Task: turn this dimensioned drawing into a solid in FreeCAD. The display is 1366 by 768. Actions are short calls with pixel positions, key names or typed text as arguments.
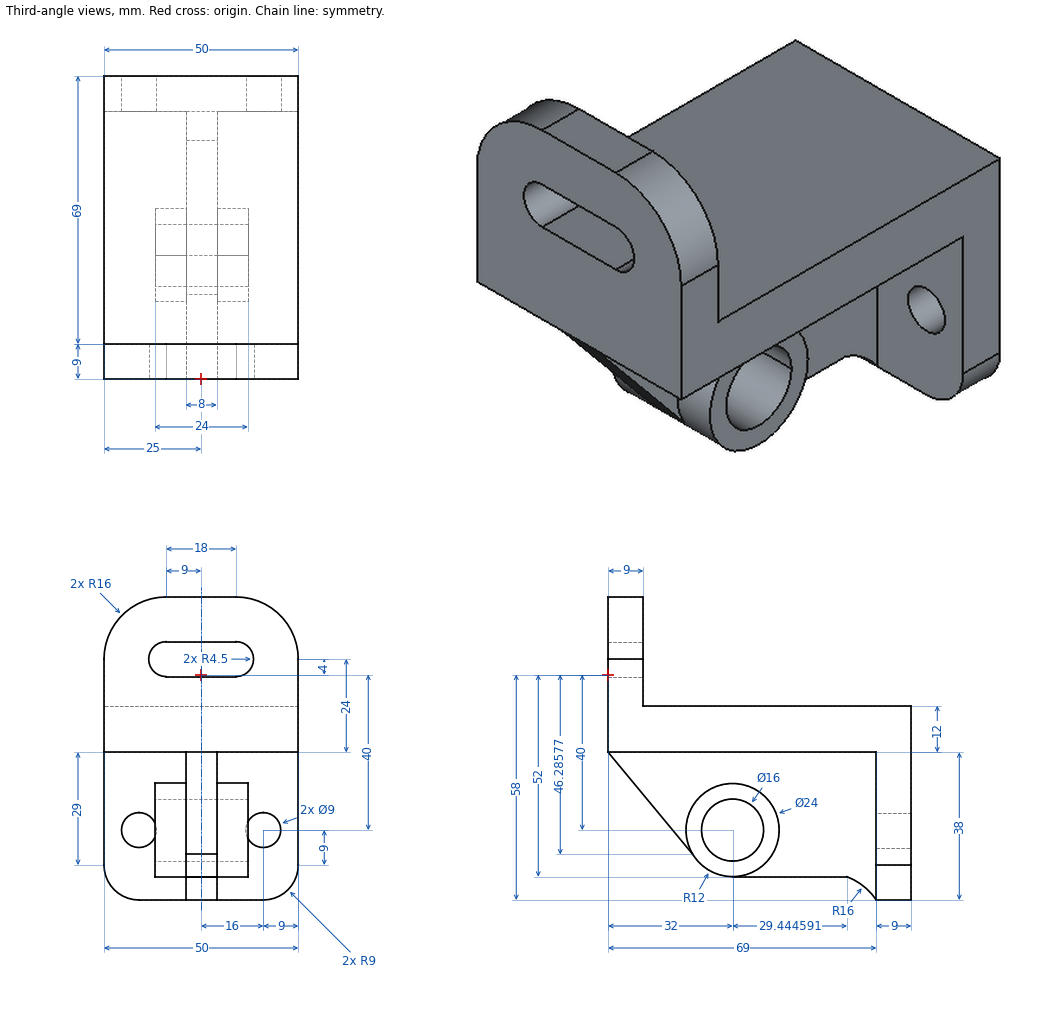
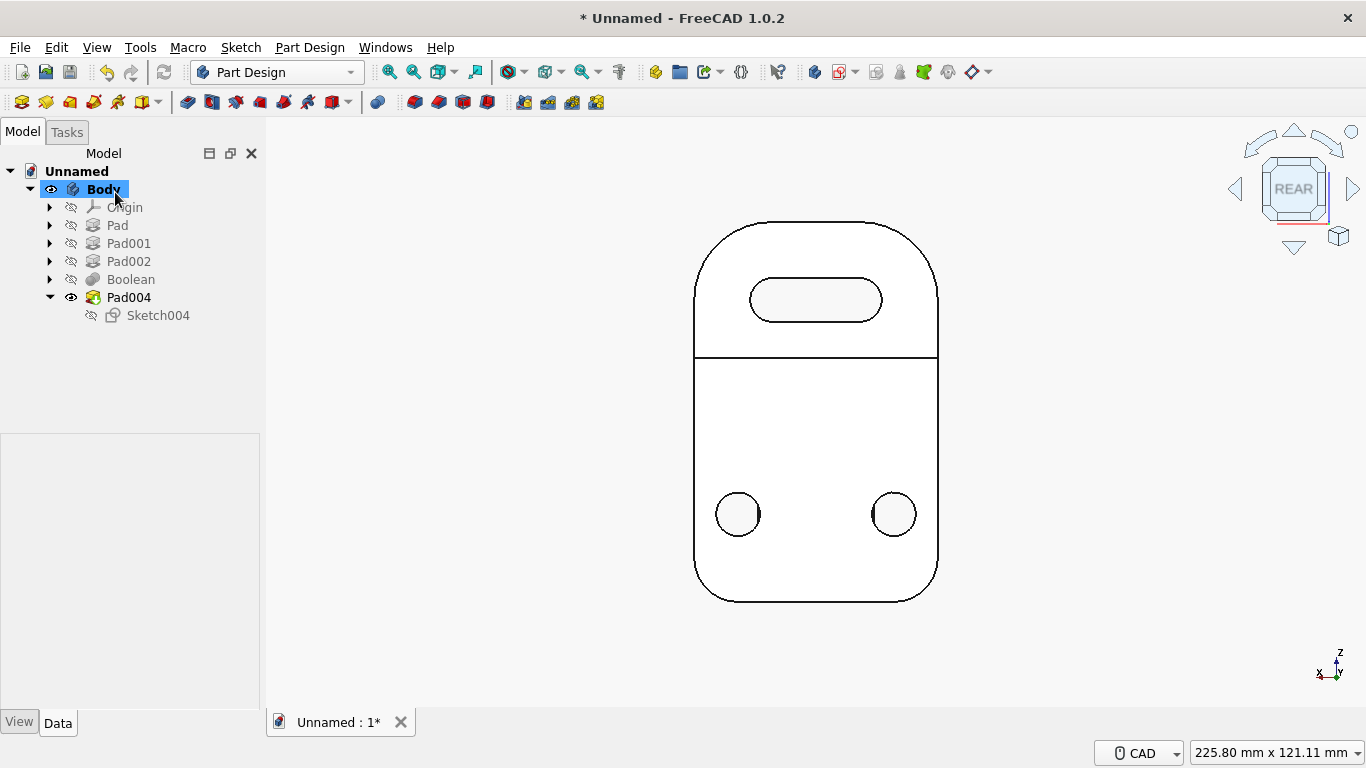
key(6)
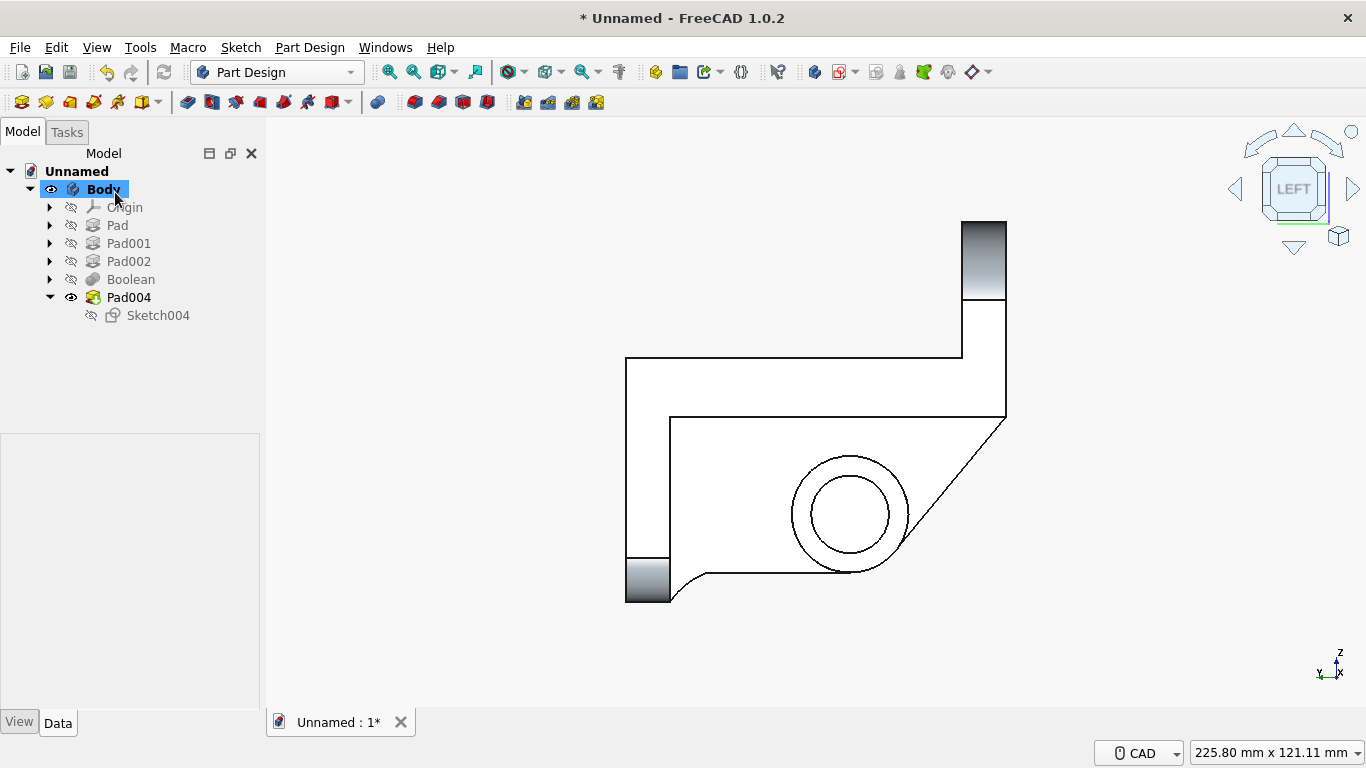
click(742, 482)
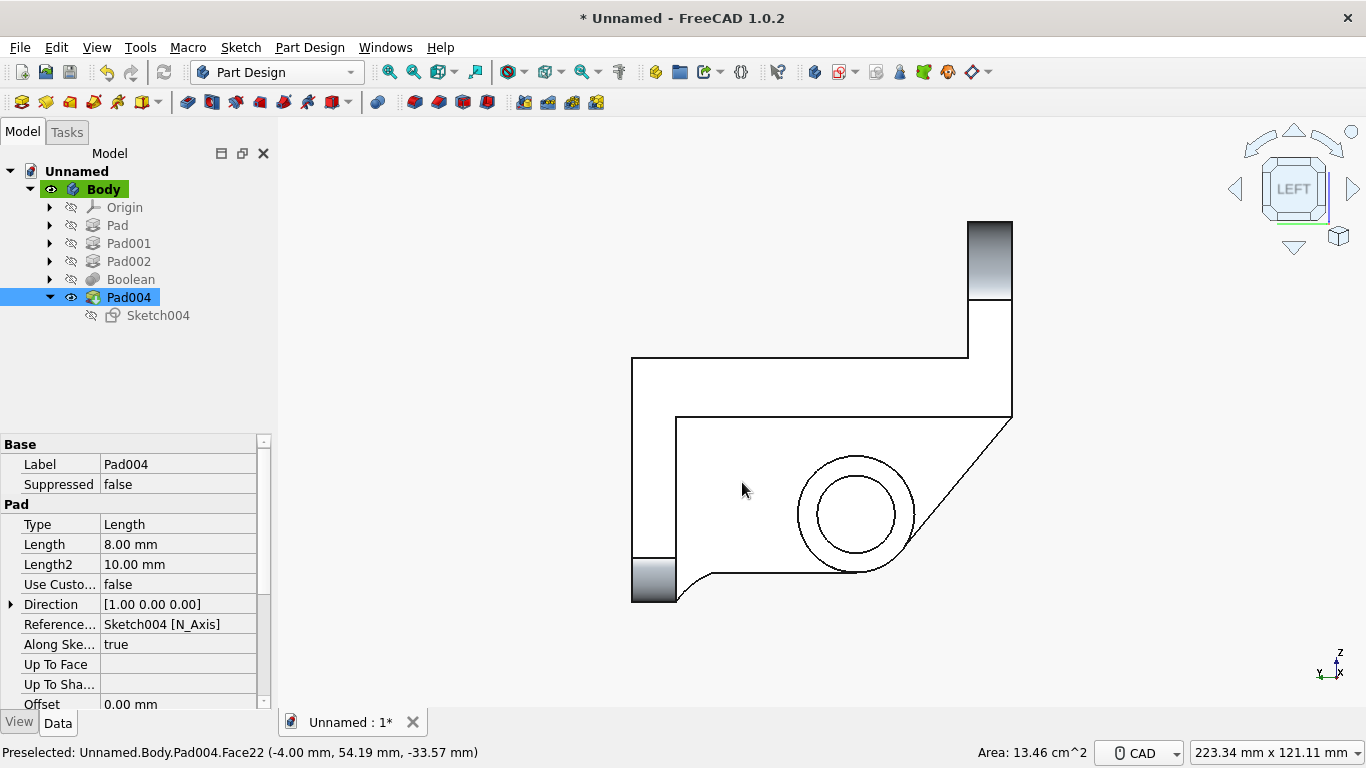
click(840, 72)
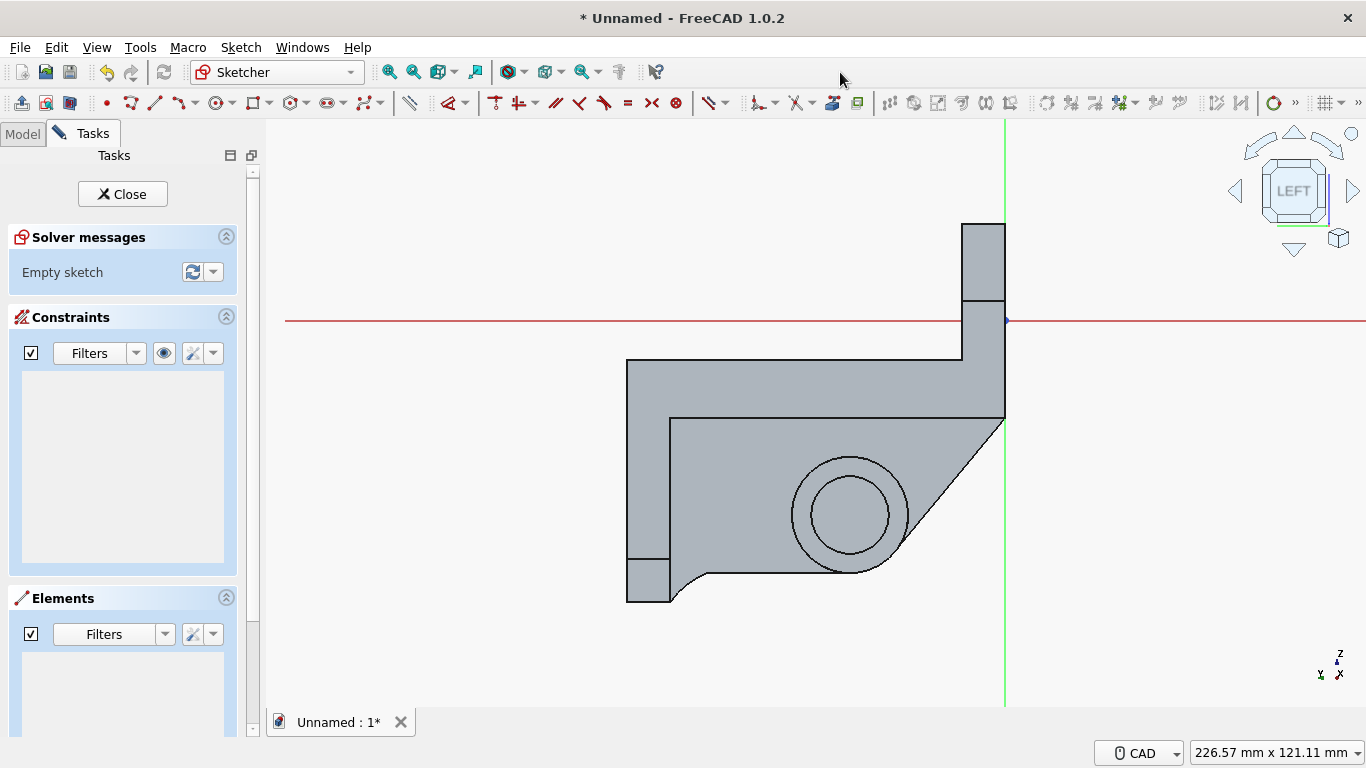
click(70, 104)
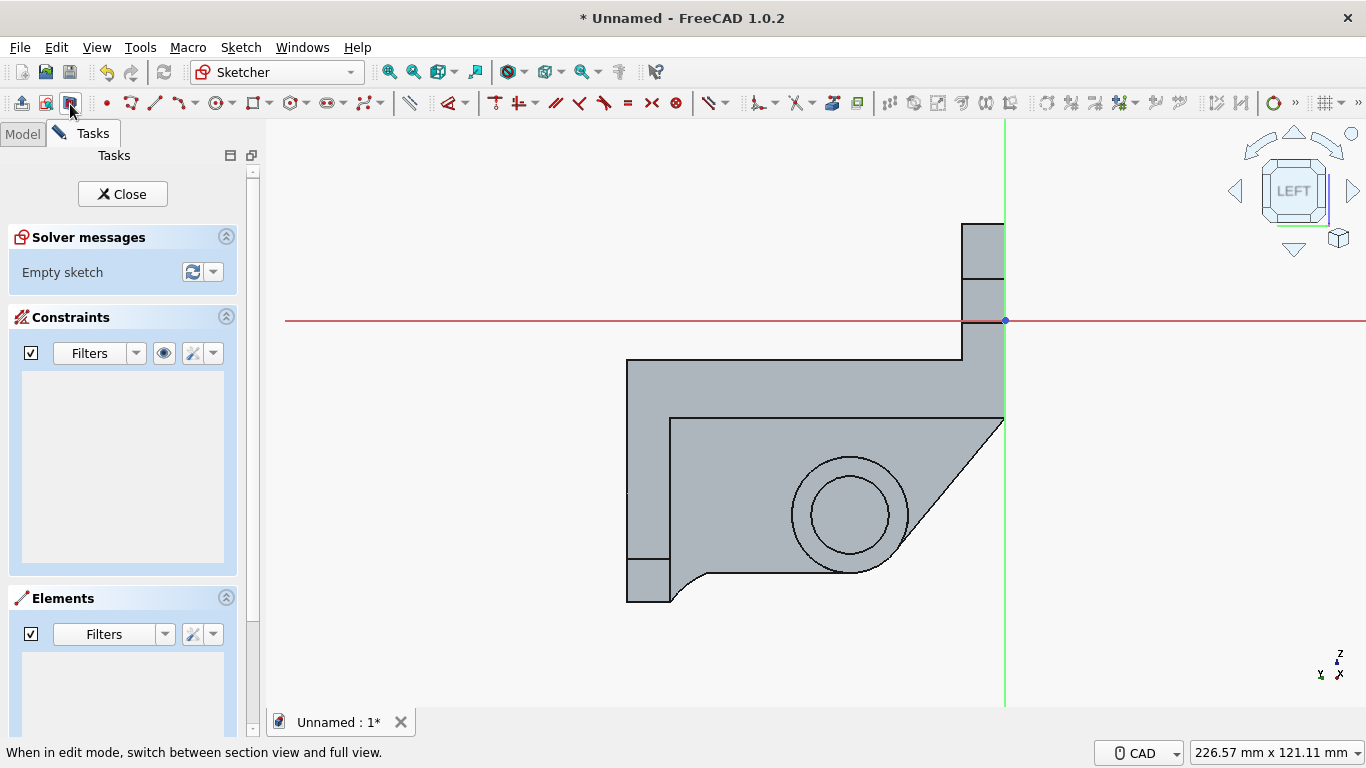
scroll(876, 541, up, 8)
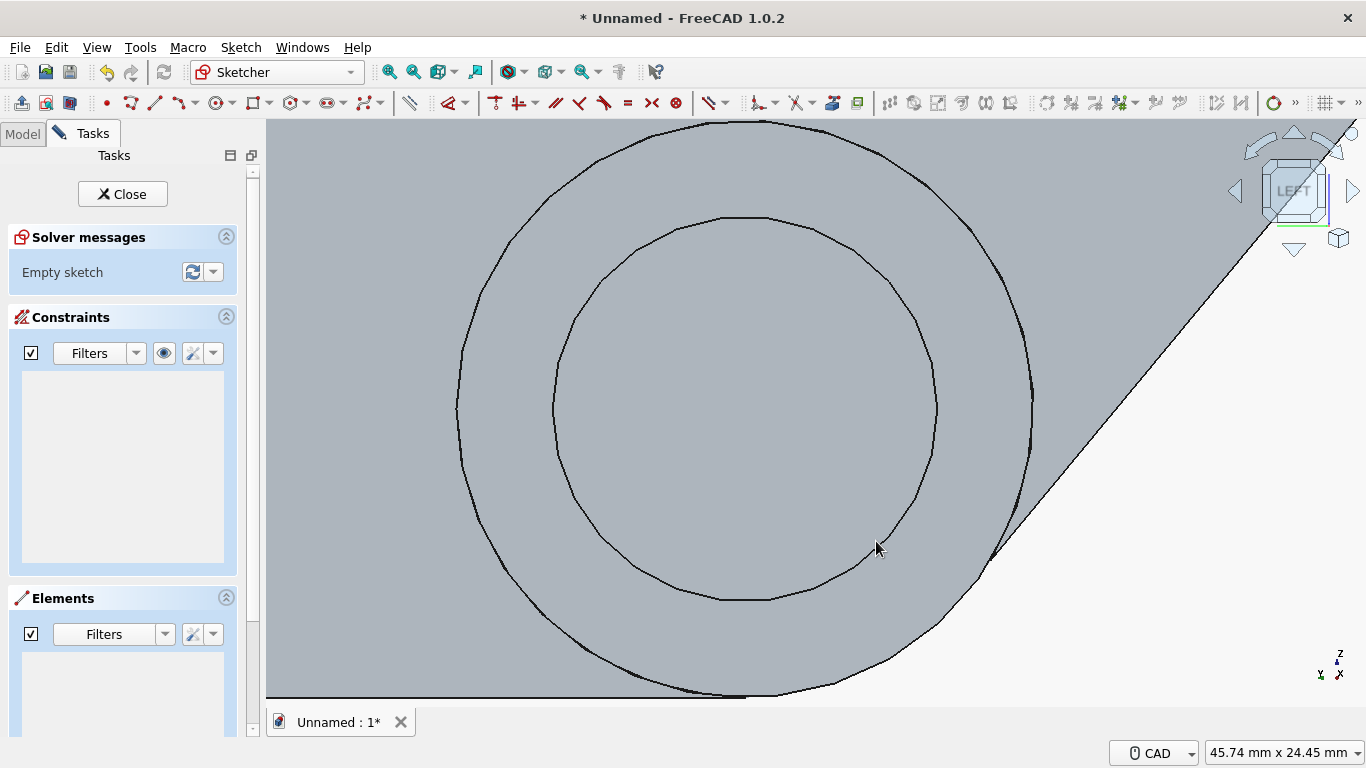
click(216, 104)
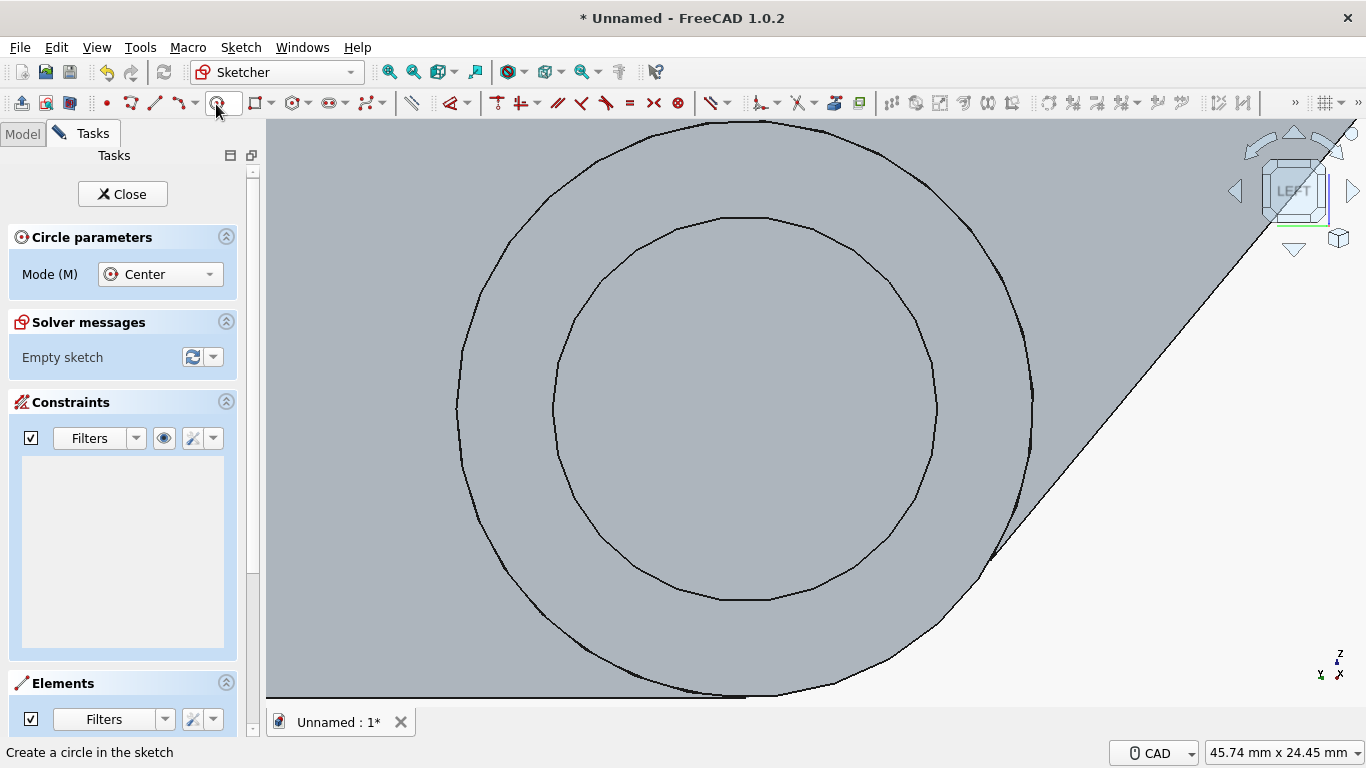
click(745, 409)
click(881, 273)
key(Escape)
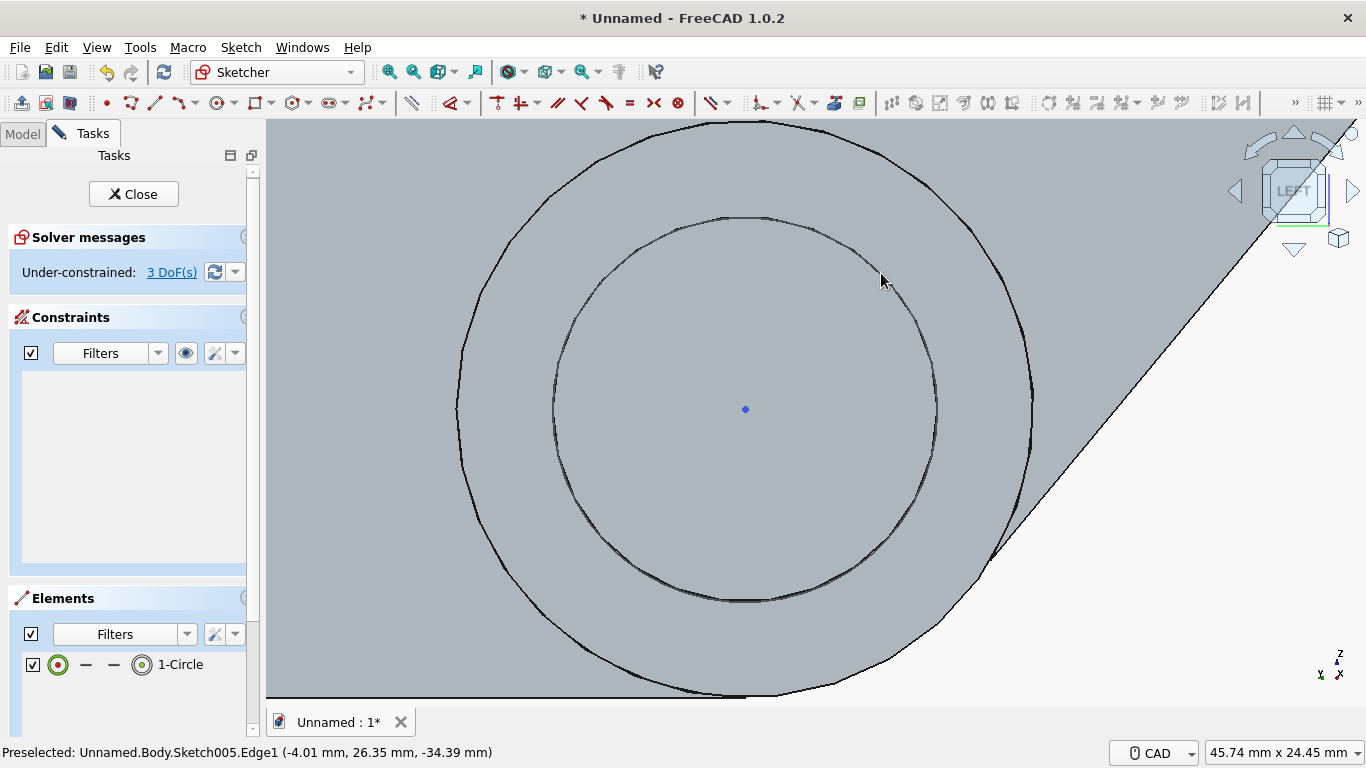
click(450, 104)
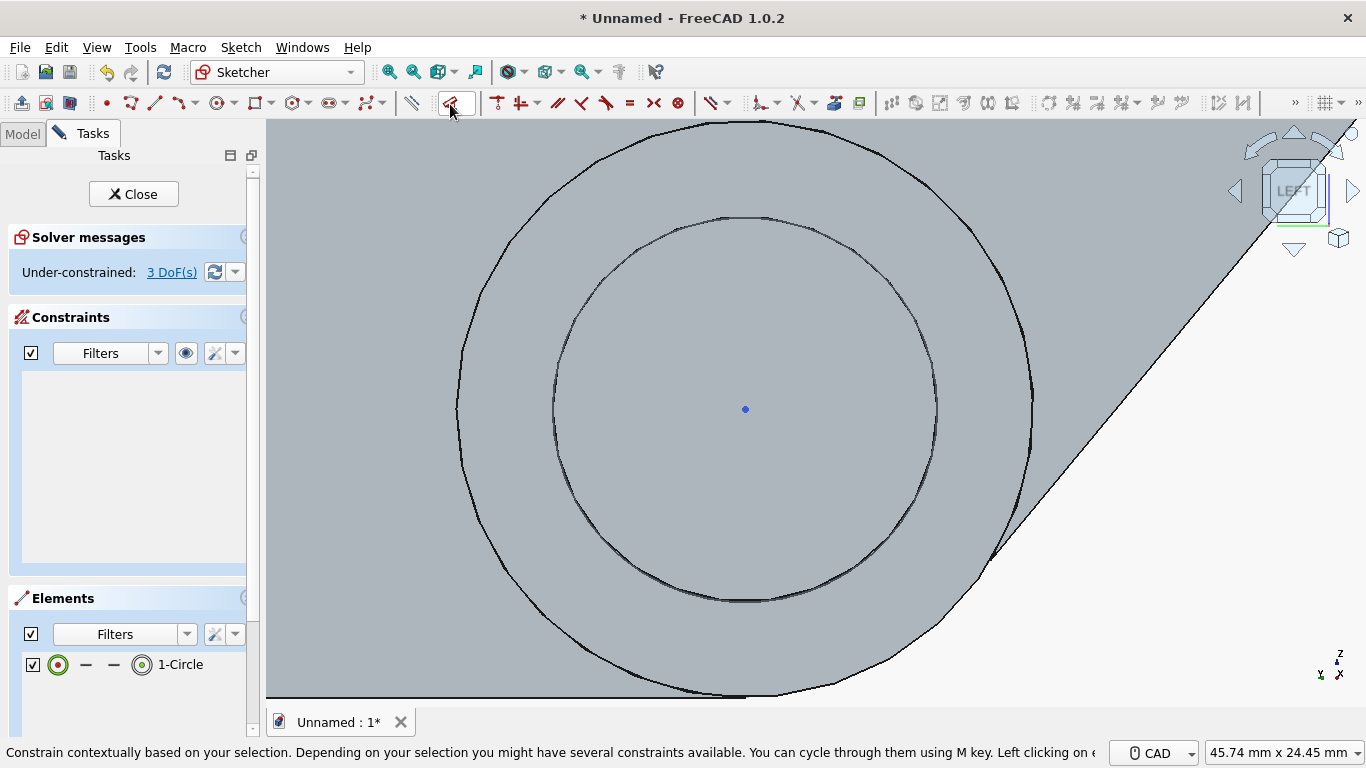
click(881, 274)
click(904, 251)